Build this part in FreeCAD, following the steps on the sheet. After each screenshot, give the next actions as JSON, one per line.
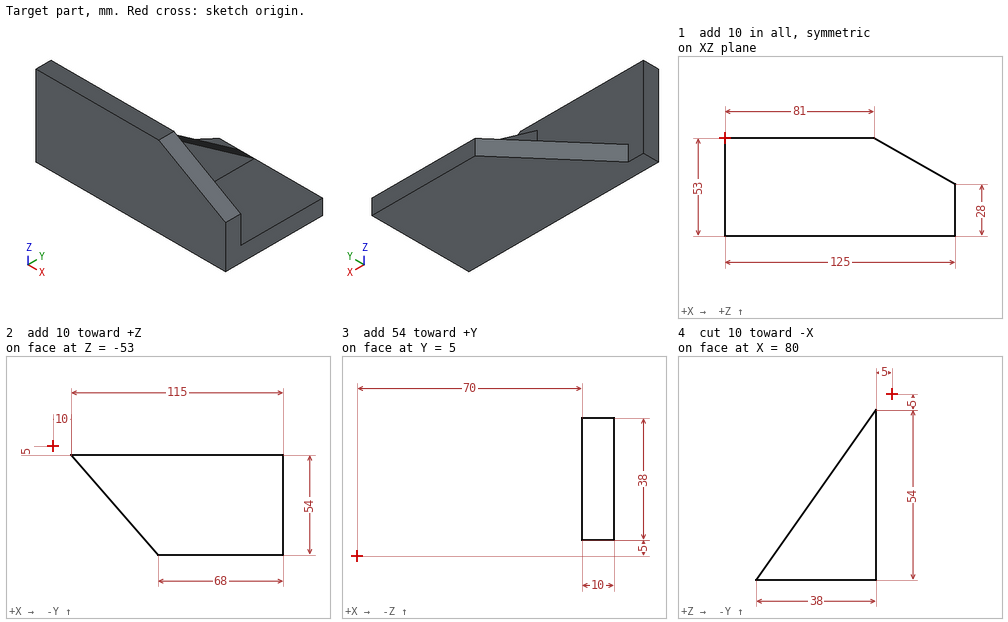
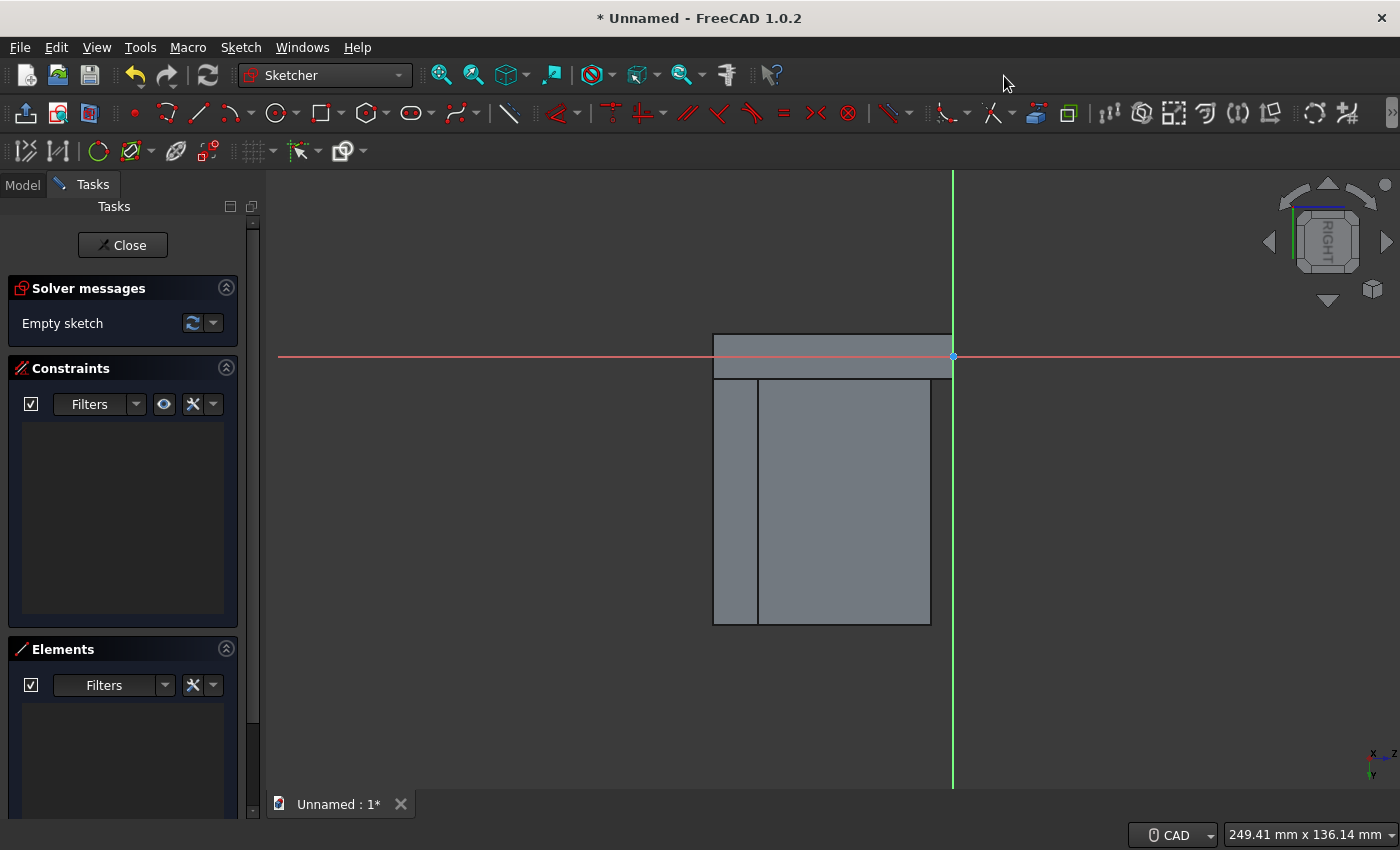
{"action": "scroll", "coordinate": [1041, 514], "scroll_direction": "up", "scroll_amount": 2}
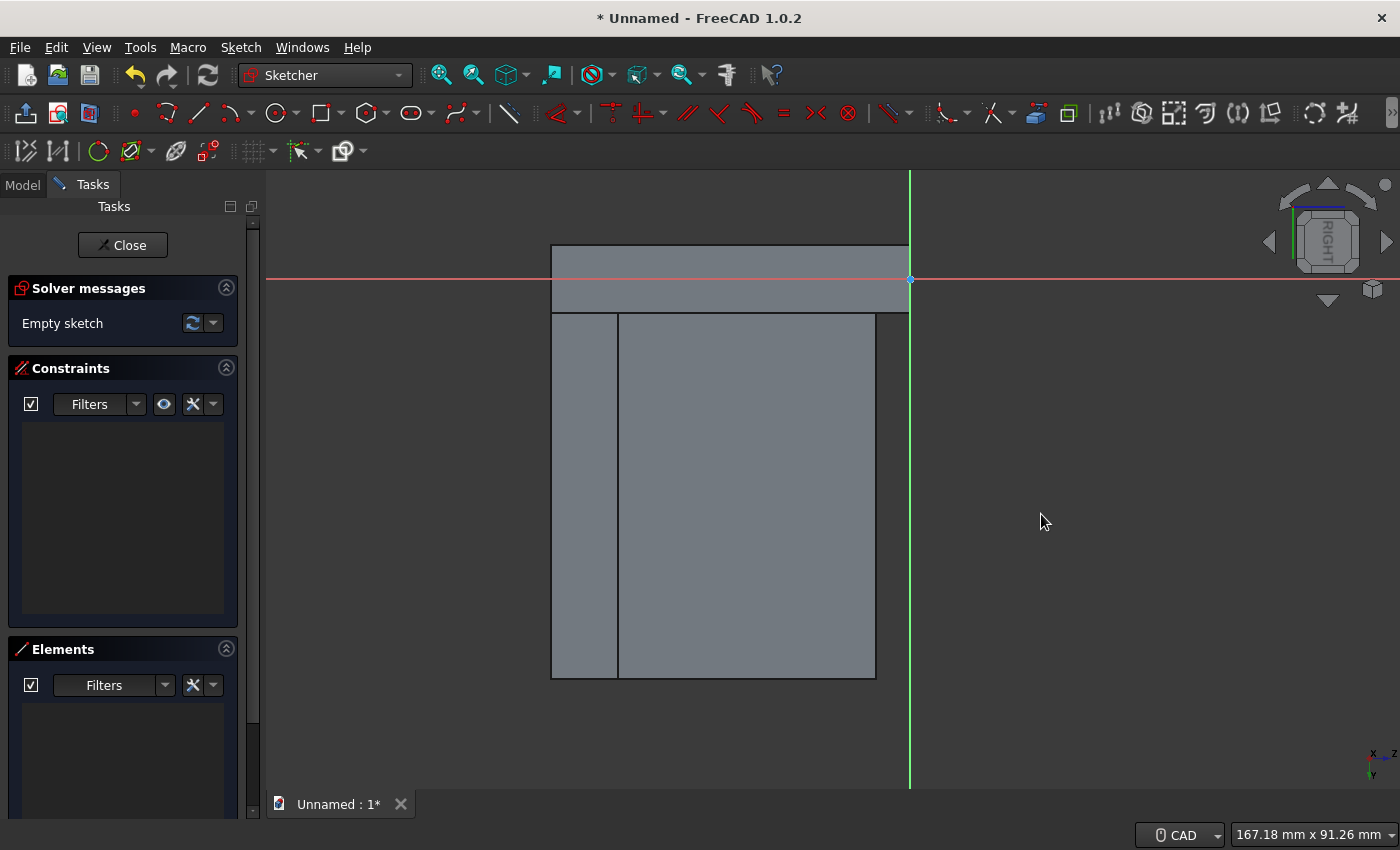
{"action": "key", "text": "g m"}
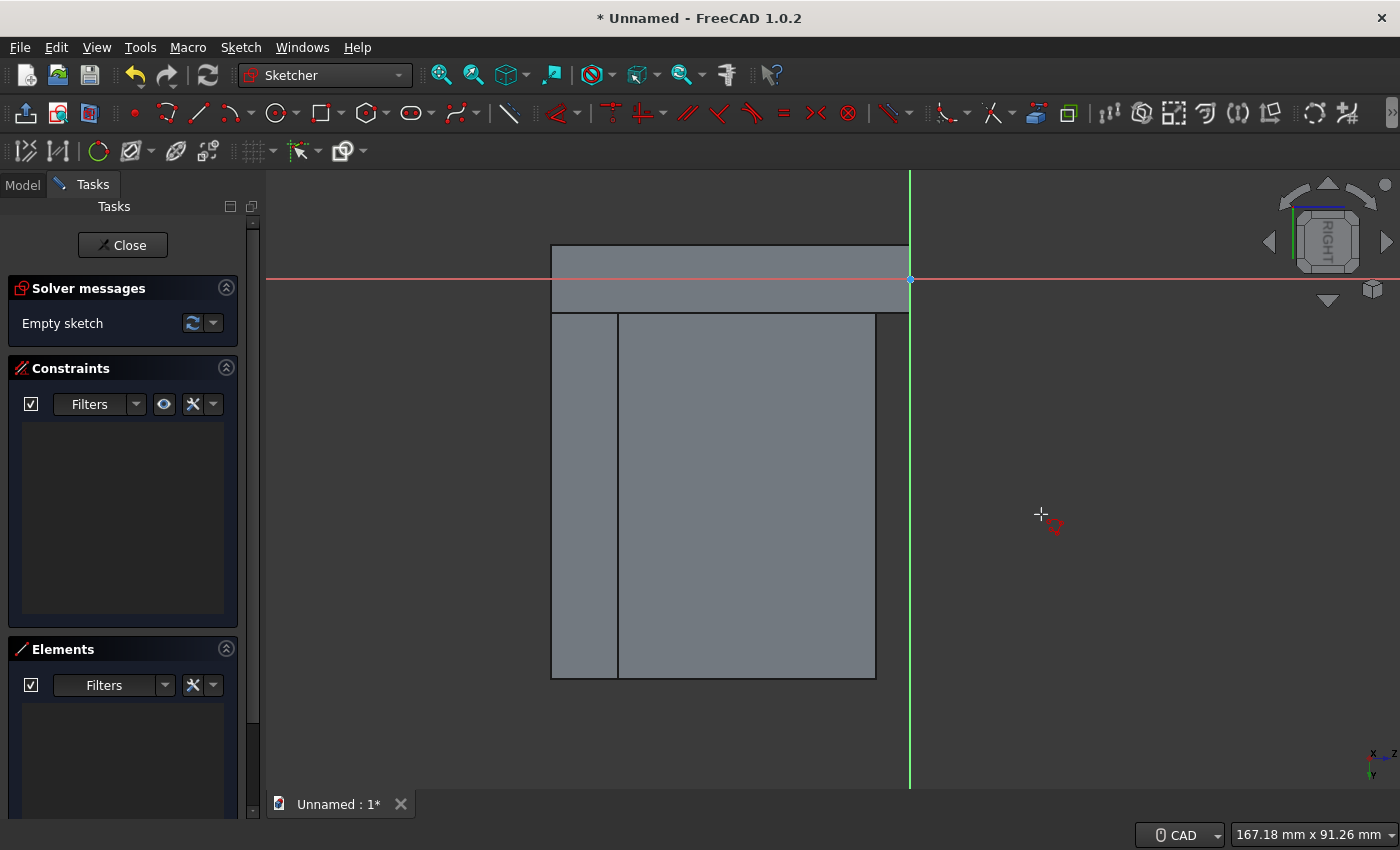
{"action": "left_click", "coordinate": [876, 313]}
{"action": "left_click", "coordinate": [618, 679]}
{"action": "left_click", "coordinate": [876, 679]}
{"action": "left_click", "coordinate": [876, 314]}
{"action": "key", "text": "Escape"}
{"action": "key", "text": "Escape"}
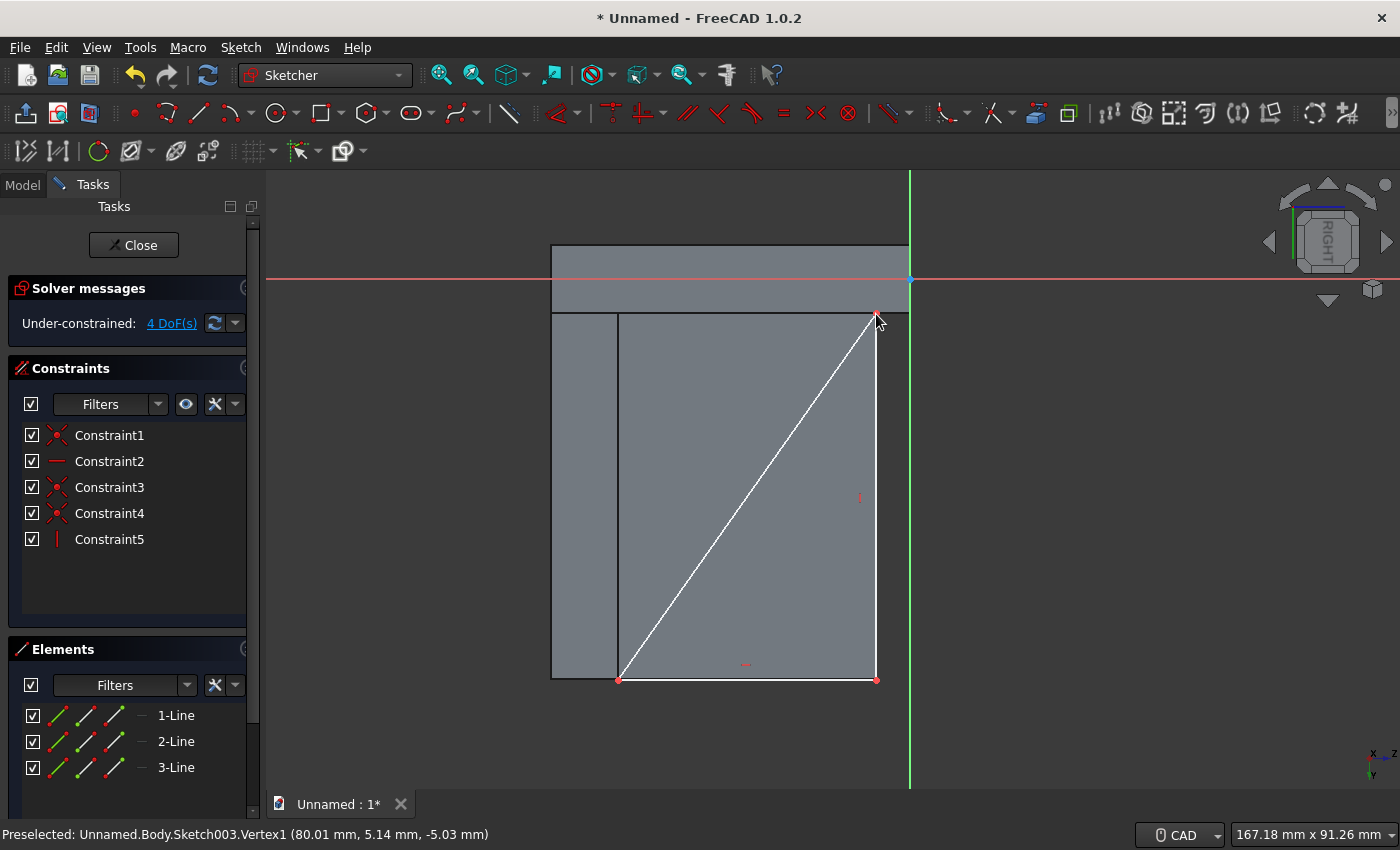
{"action": "key", "text": "d"}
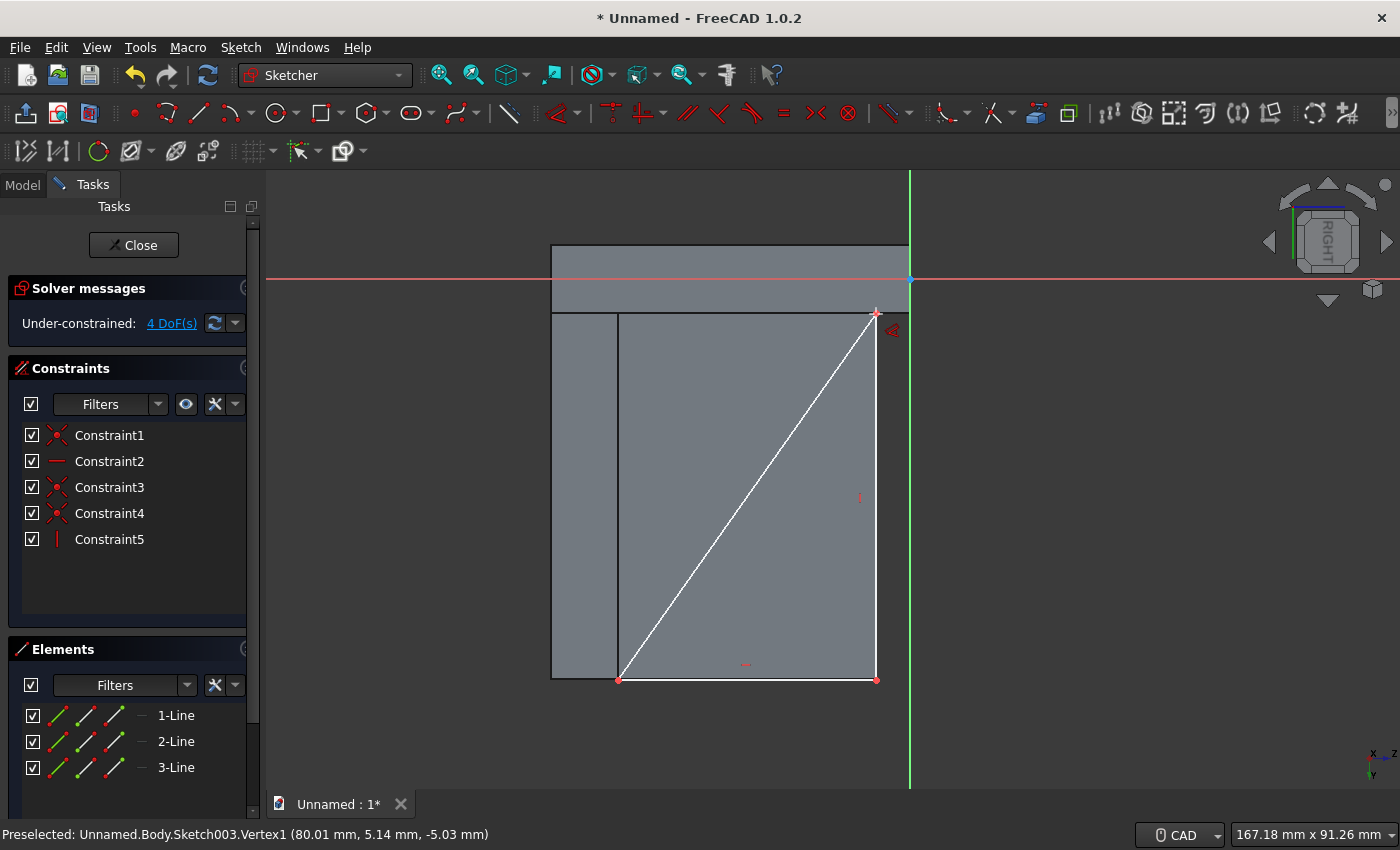
{"action": "left_click", "coordinate": [695, 680]}
{"action": "left_click", "coordinate": [747, 714]}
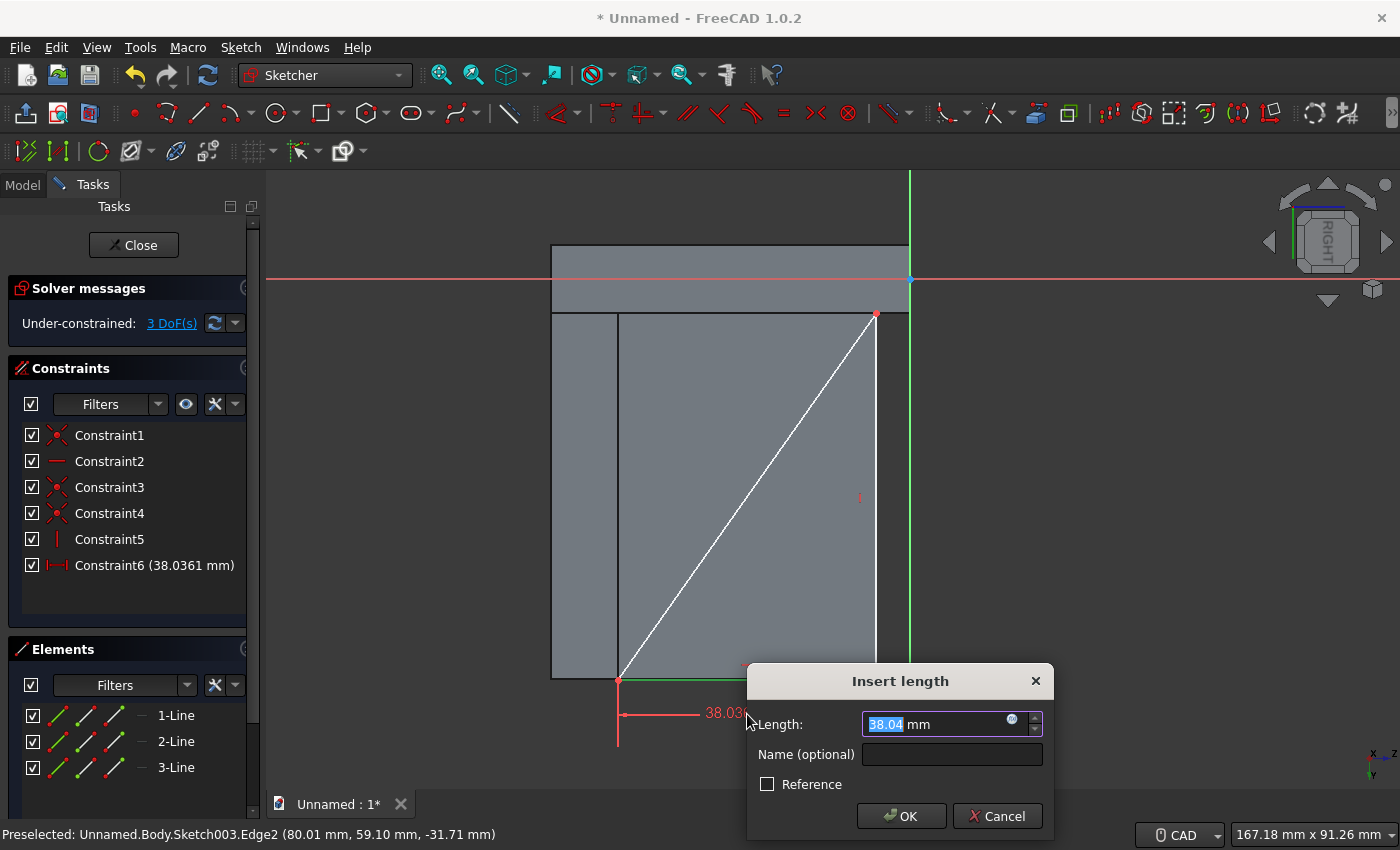
{"action": "type", "text": "38"}
{"action": "key", "text": "Return"}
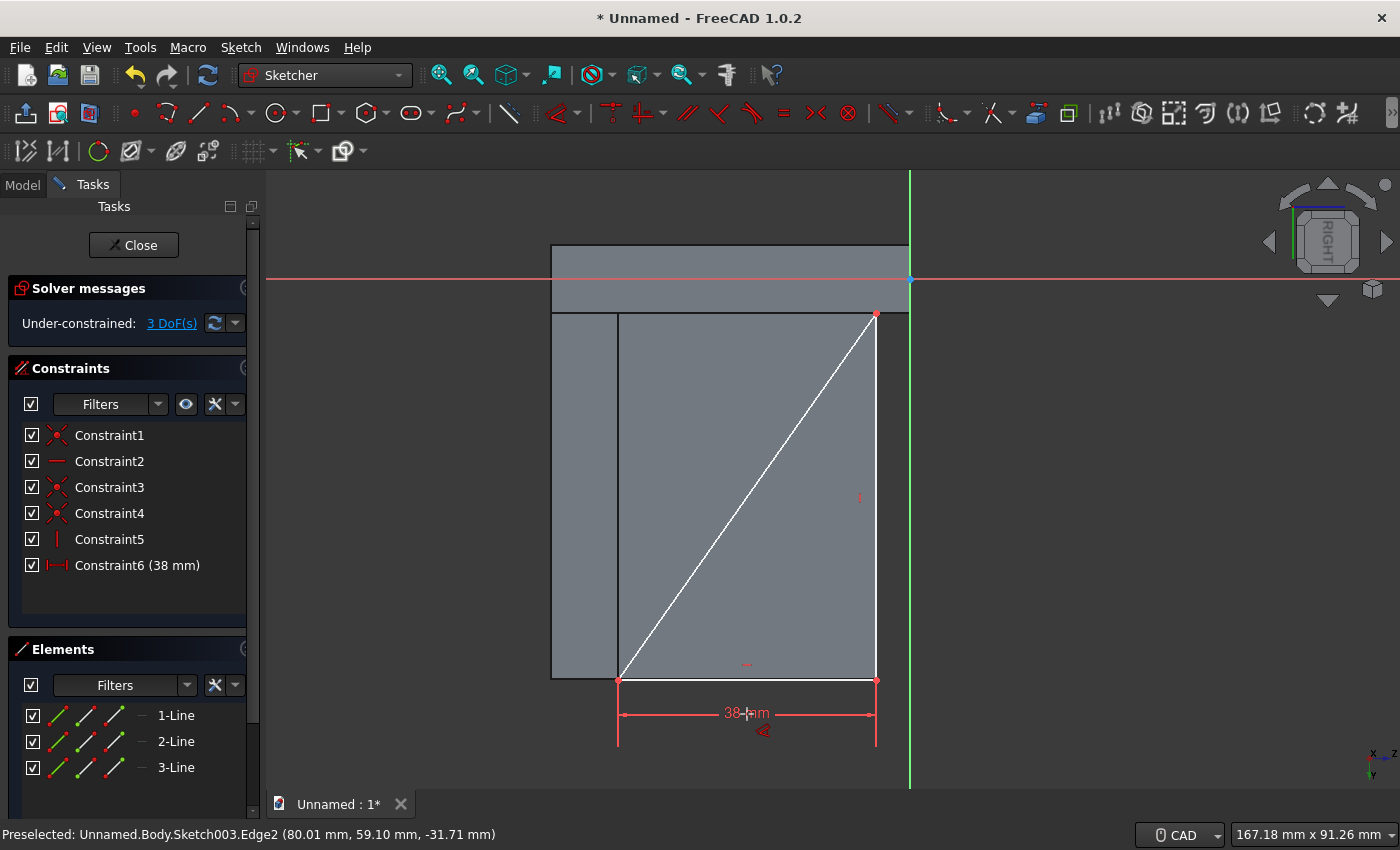
{"action": "left_click", "coordinate": [876, 570]}
{"action": "left_click", "coordinate": [842, 497]}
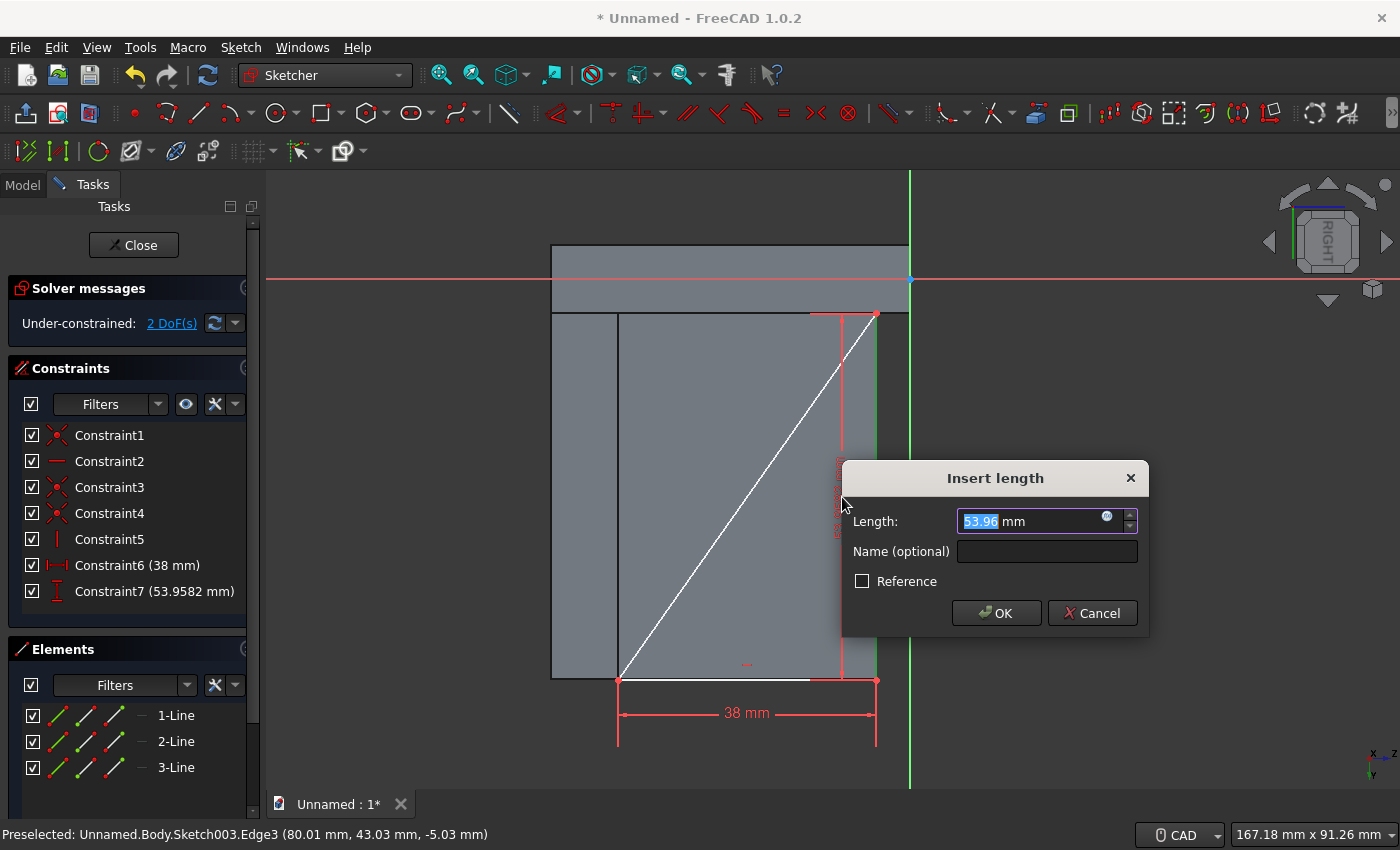
{"action": "type", "text": "54"}
{"action": "key", "text": "Return"}